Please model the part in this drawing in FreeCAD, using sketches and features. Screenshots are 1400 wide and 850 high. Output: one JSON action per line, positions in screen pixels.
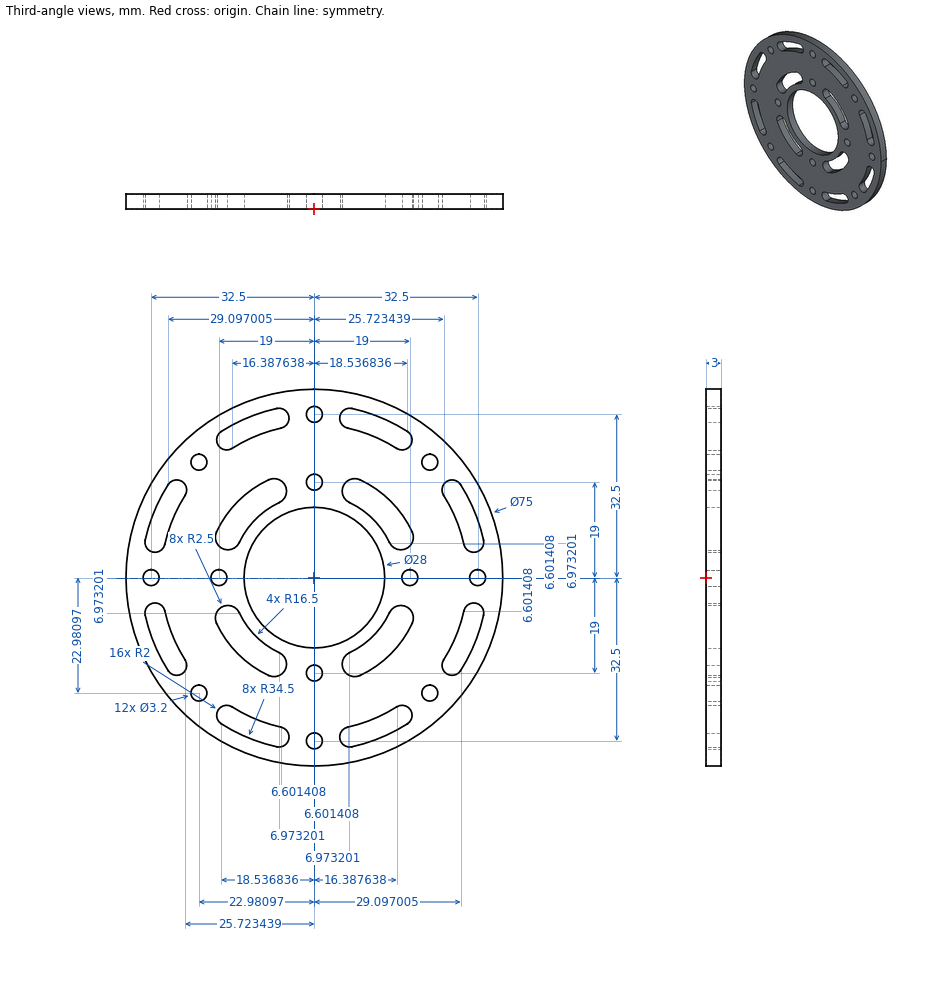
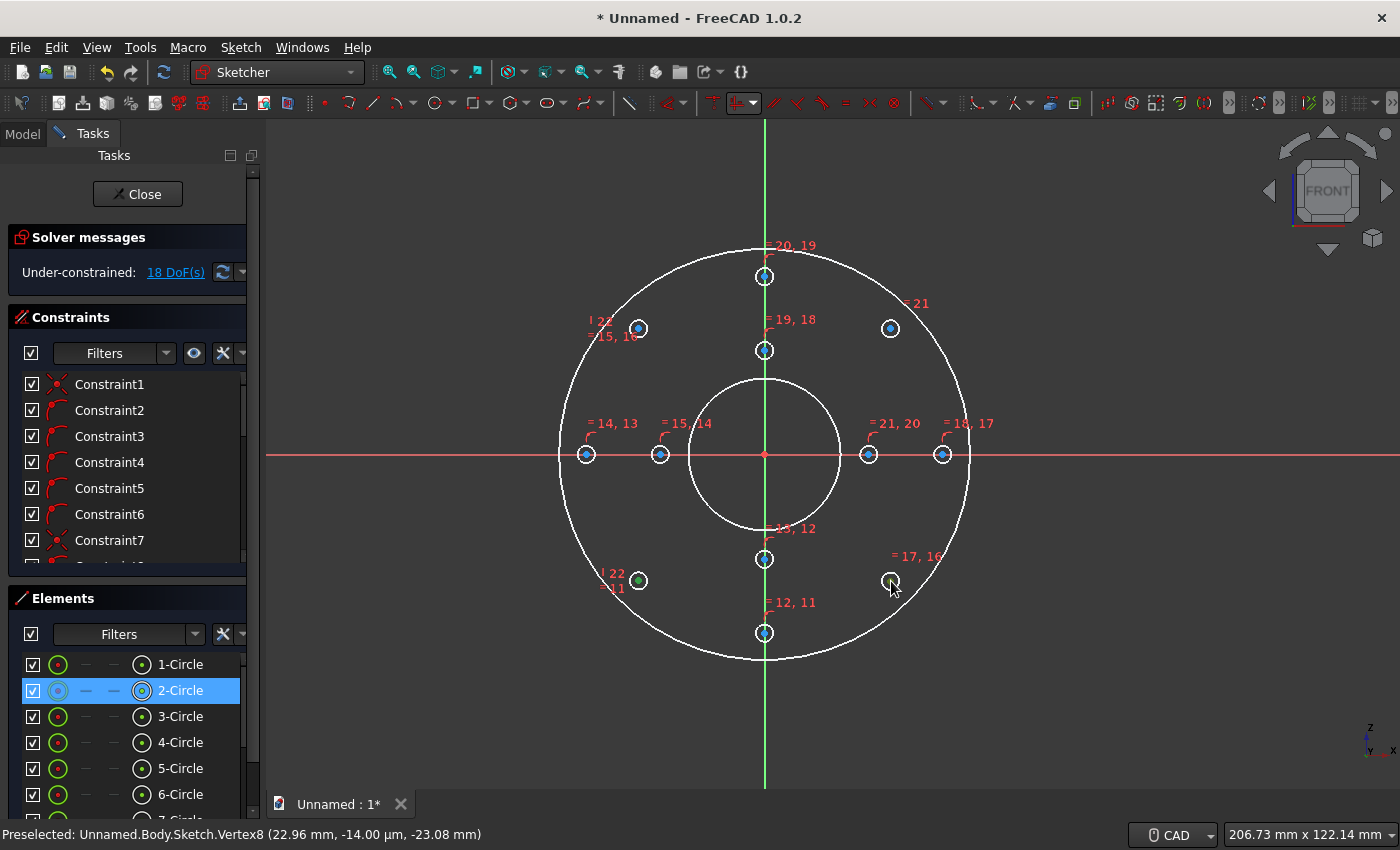
{"action": "left_click", "coordinate": [756, 104]}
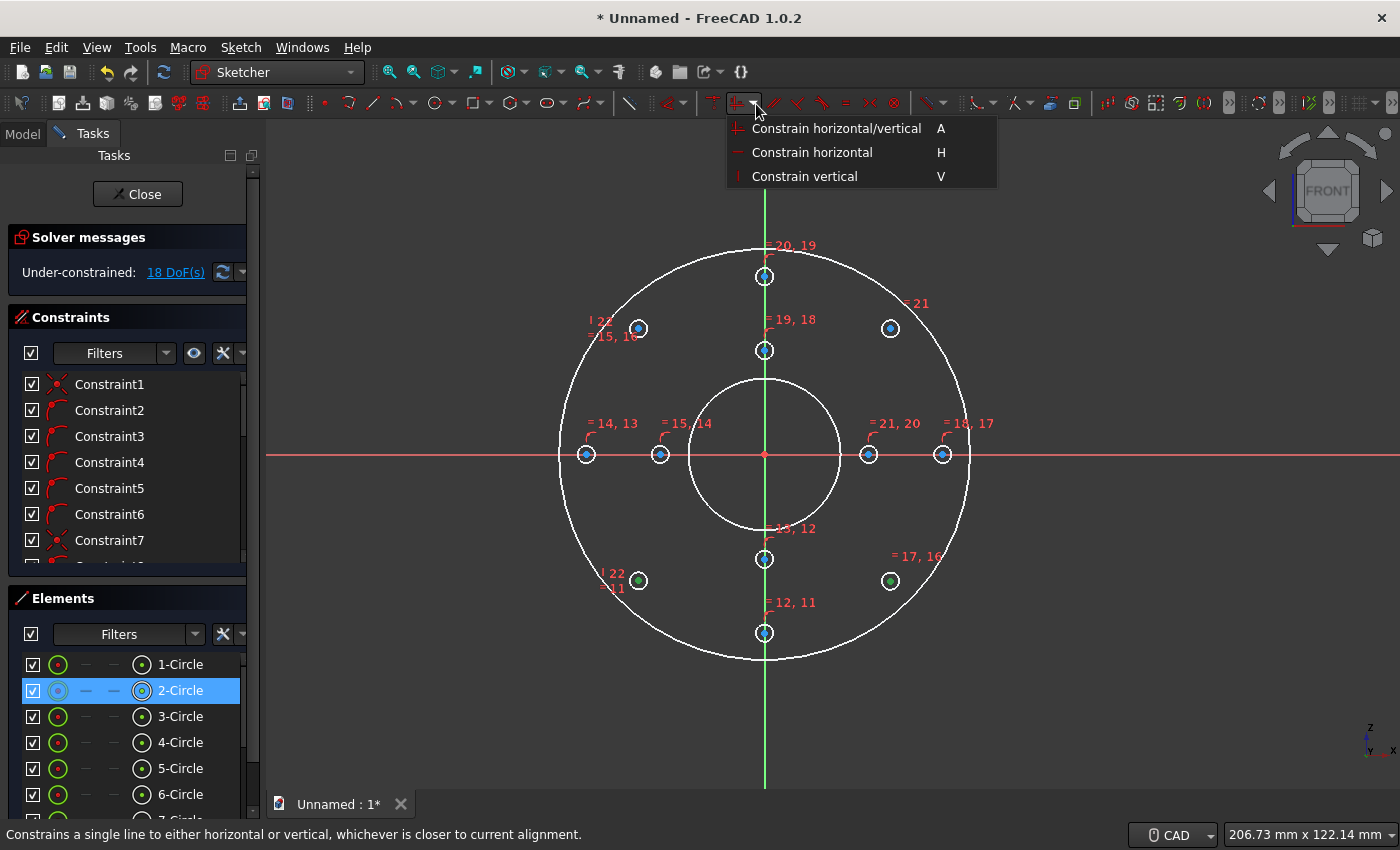
{"action": "left_click", "coordinate": [862, 152]}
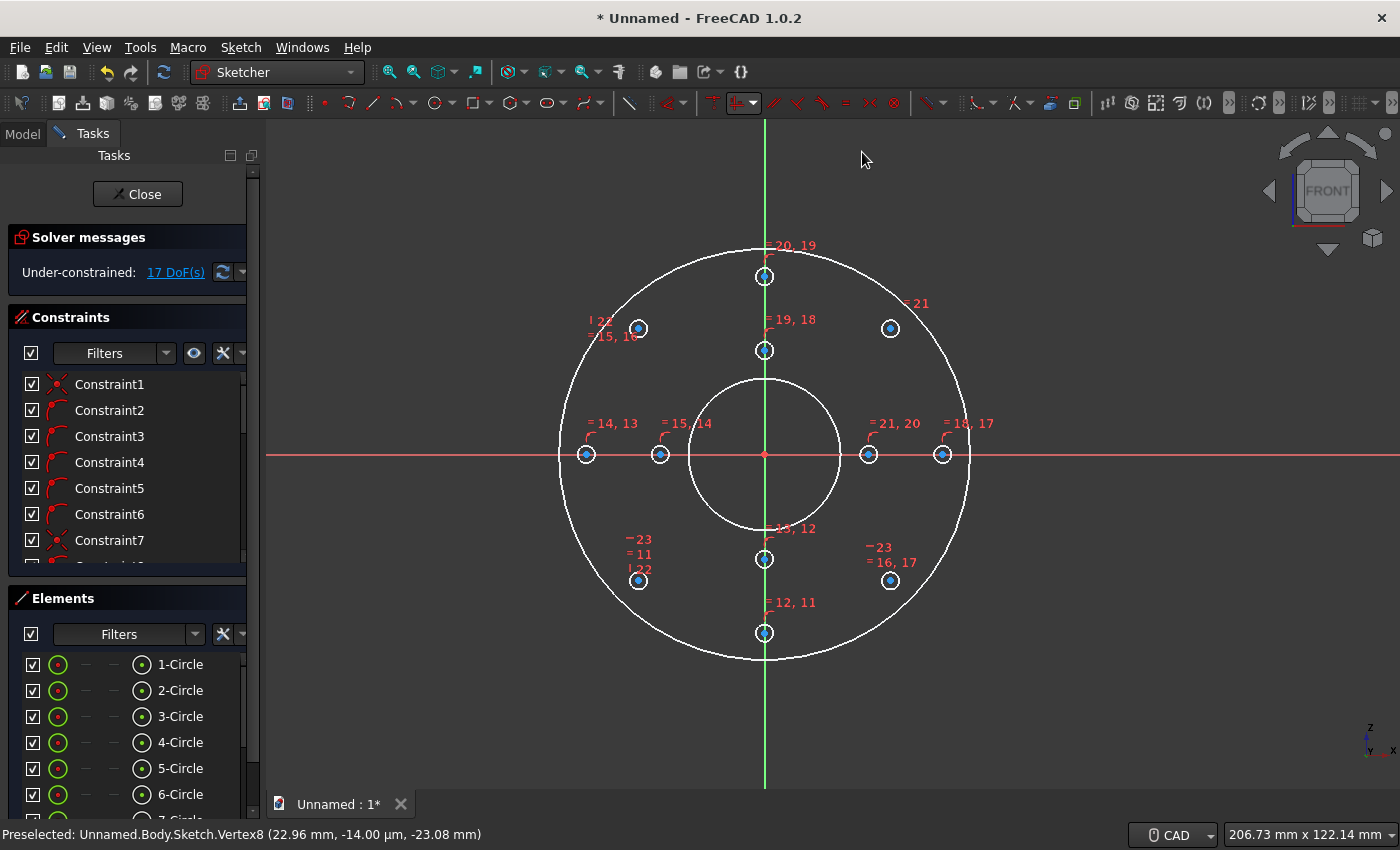
{"action": "left_click", "coordinate": [639, 329]}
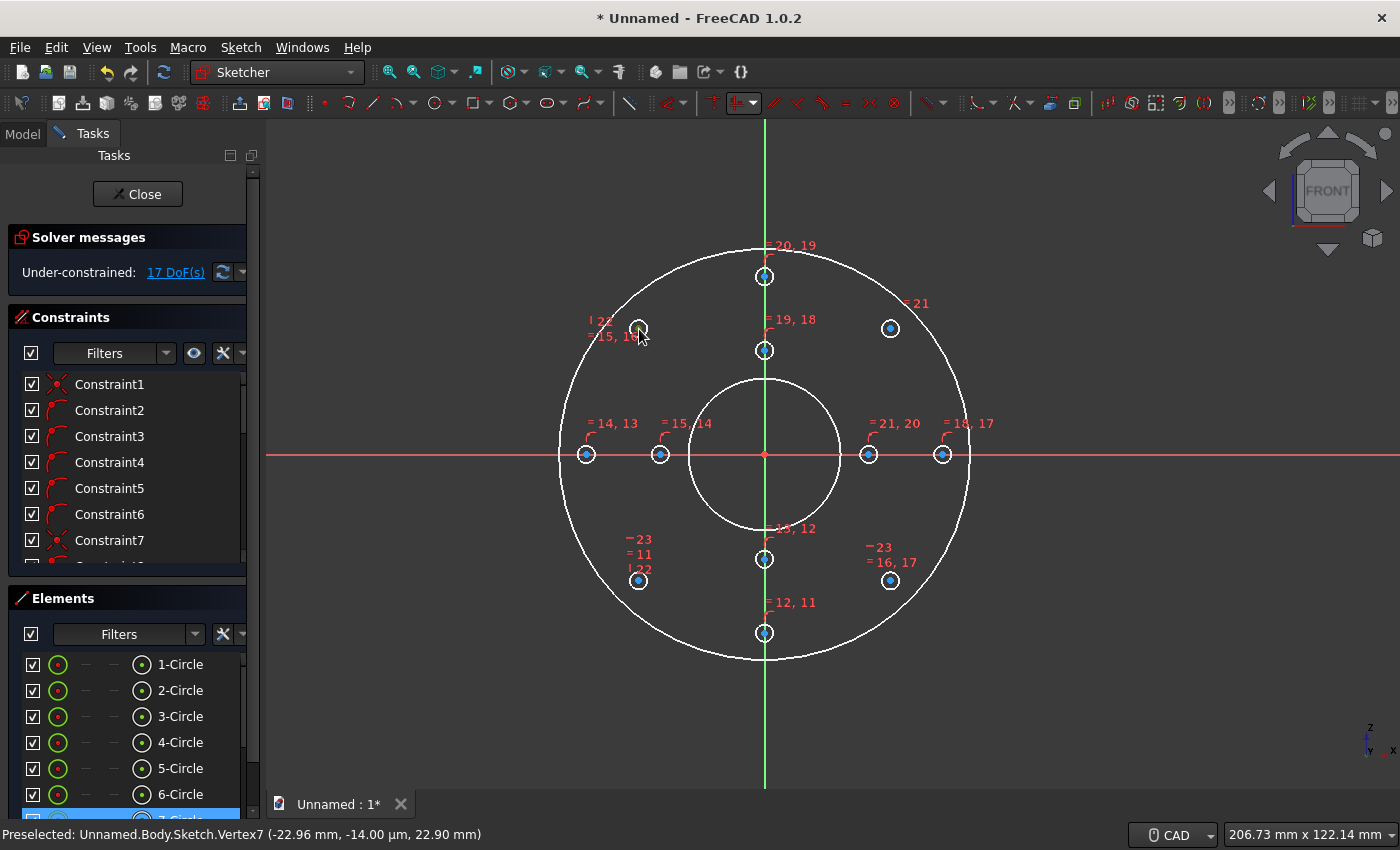
{"action": "left_click", "coordinate": [891, 329]}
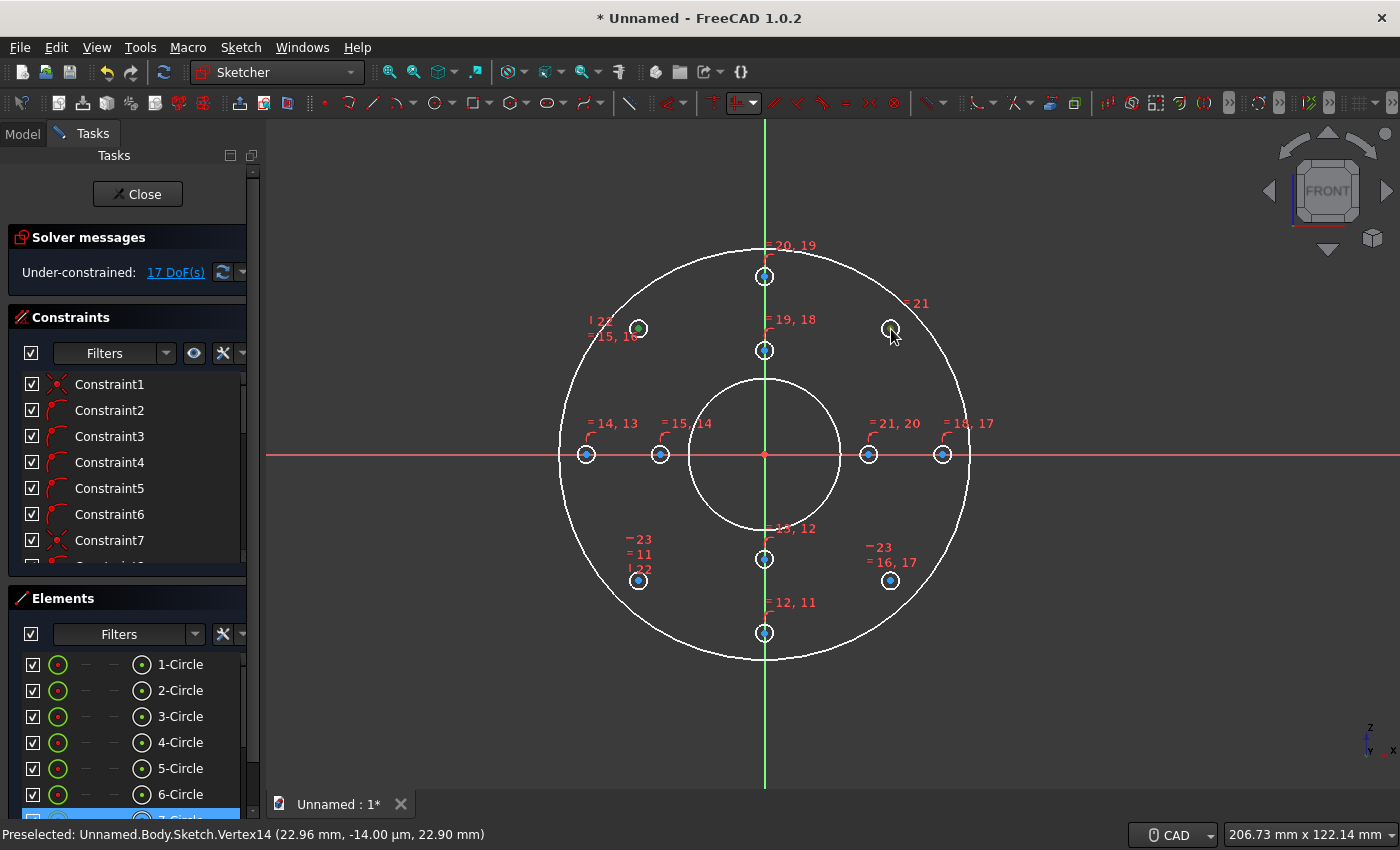
{"action": "left_click", "coordinate": [765, 717]}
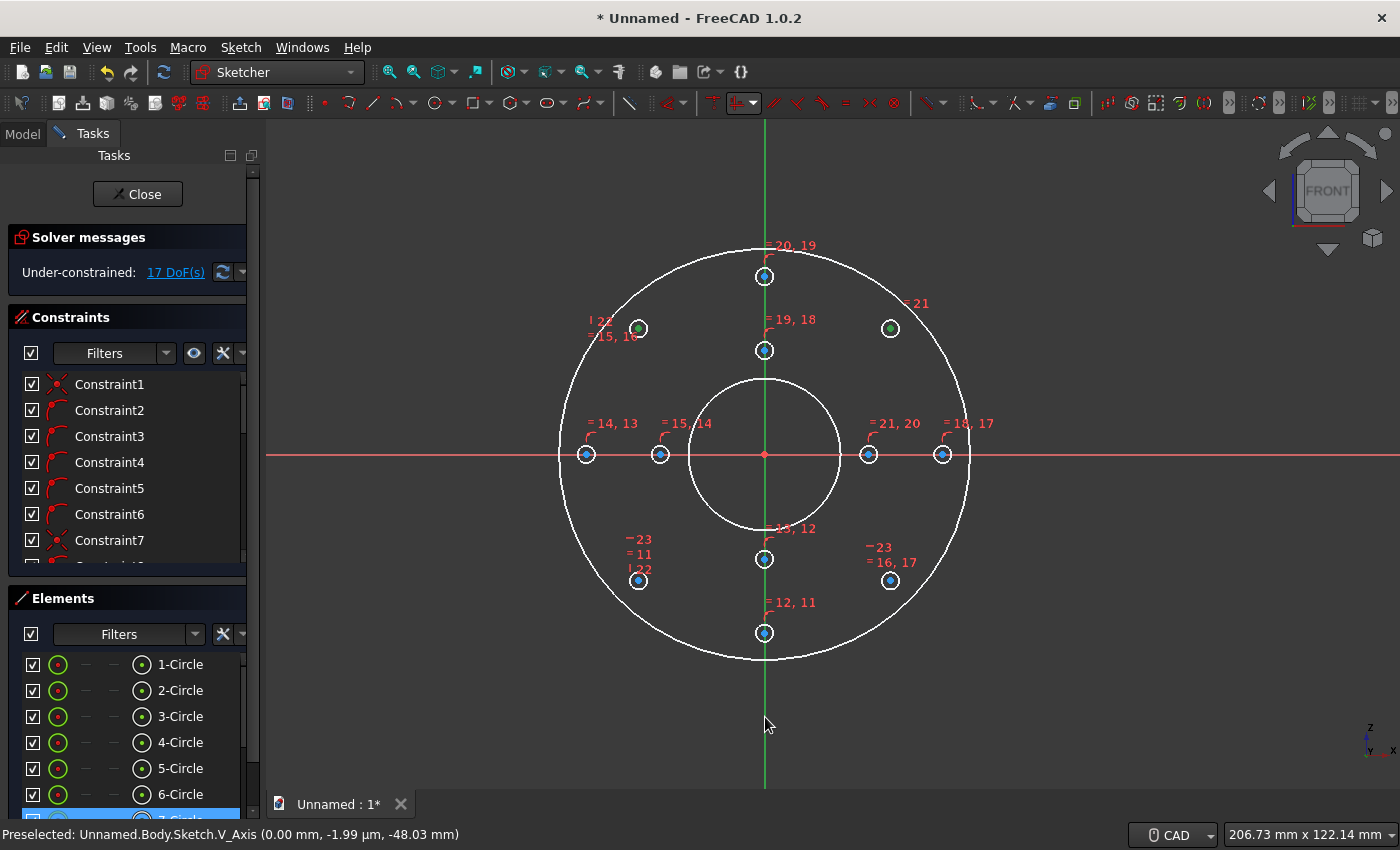
{"action": "left_click", "coordinate": [870, 104]}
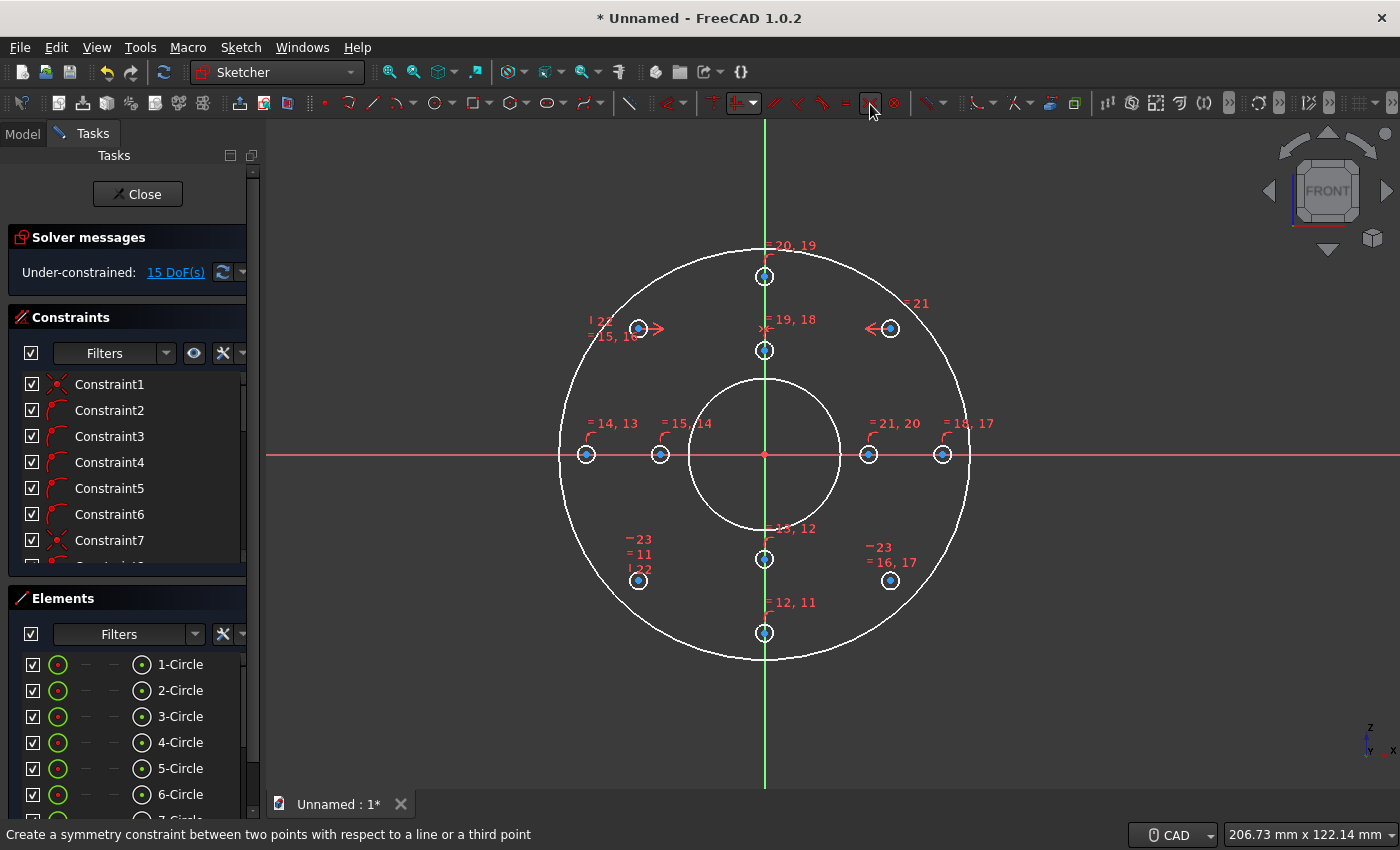
{"action": "left_click", "coordinate": [891, 581]}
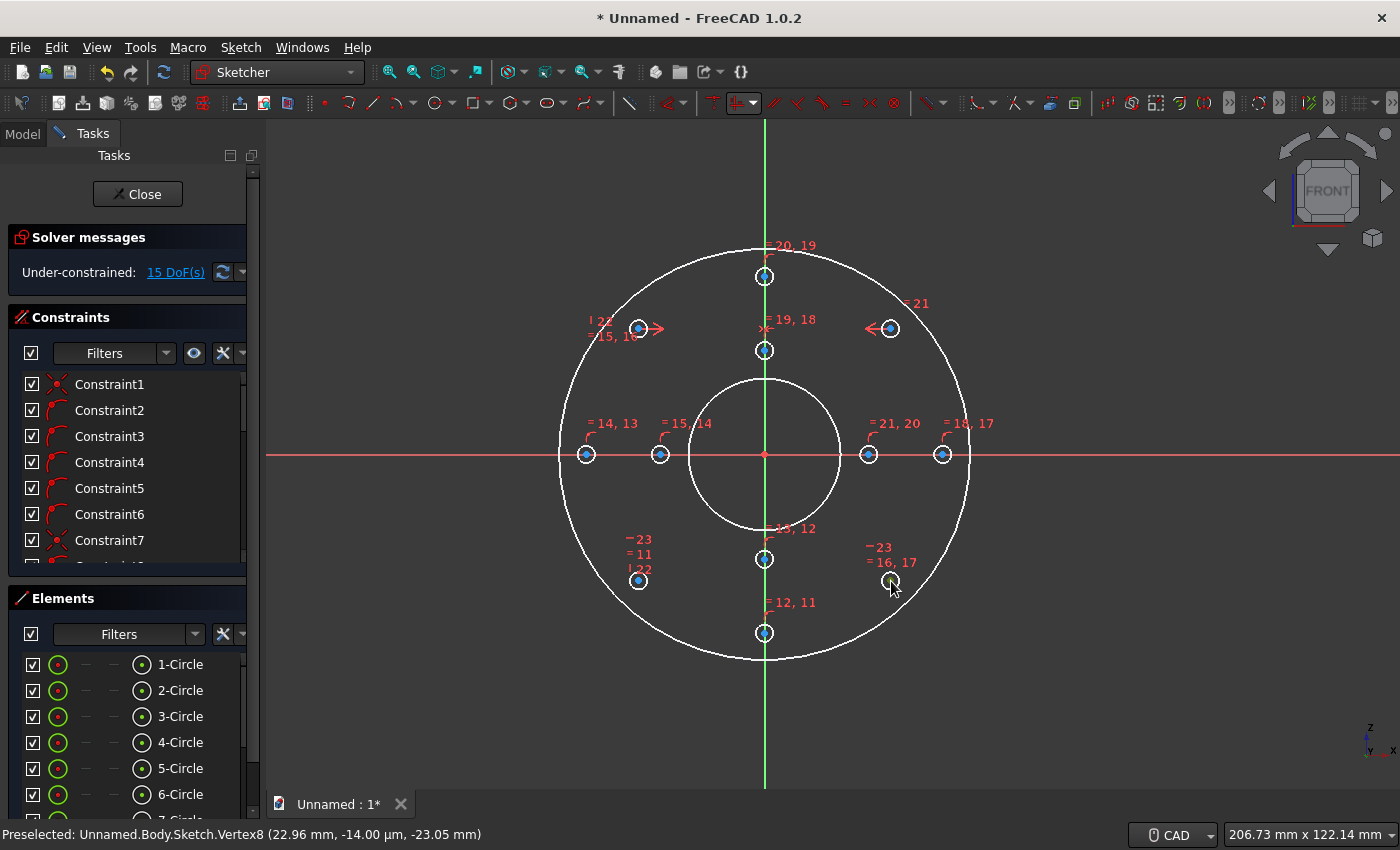
{"action": "left_click", "coordinate": [891, 329]}